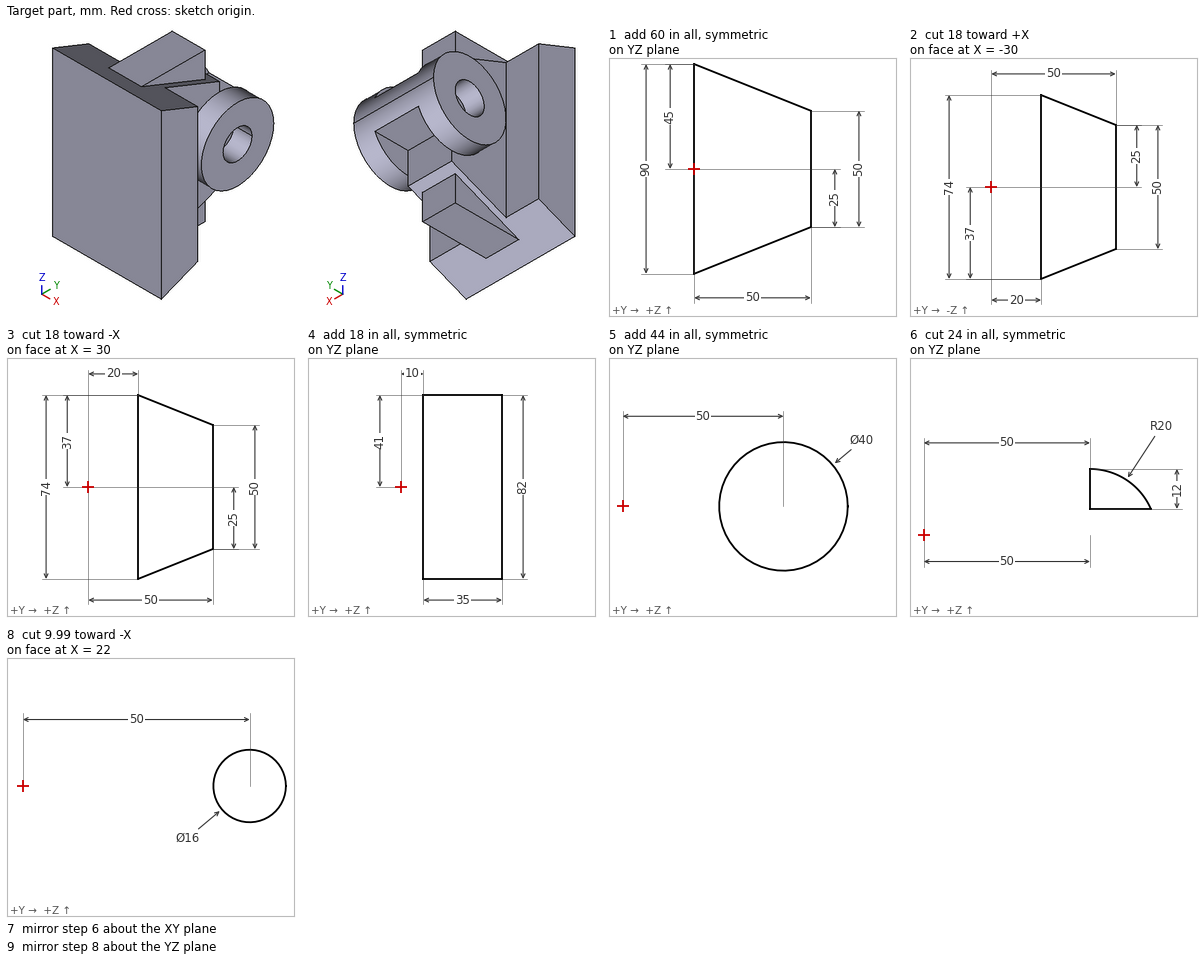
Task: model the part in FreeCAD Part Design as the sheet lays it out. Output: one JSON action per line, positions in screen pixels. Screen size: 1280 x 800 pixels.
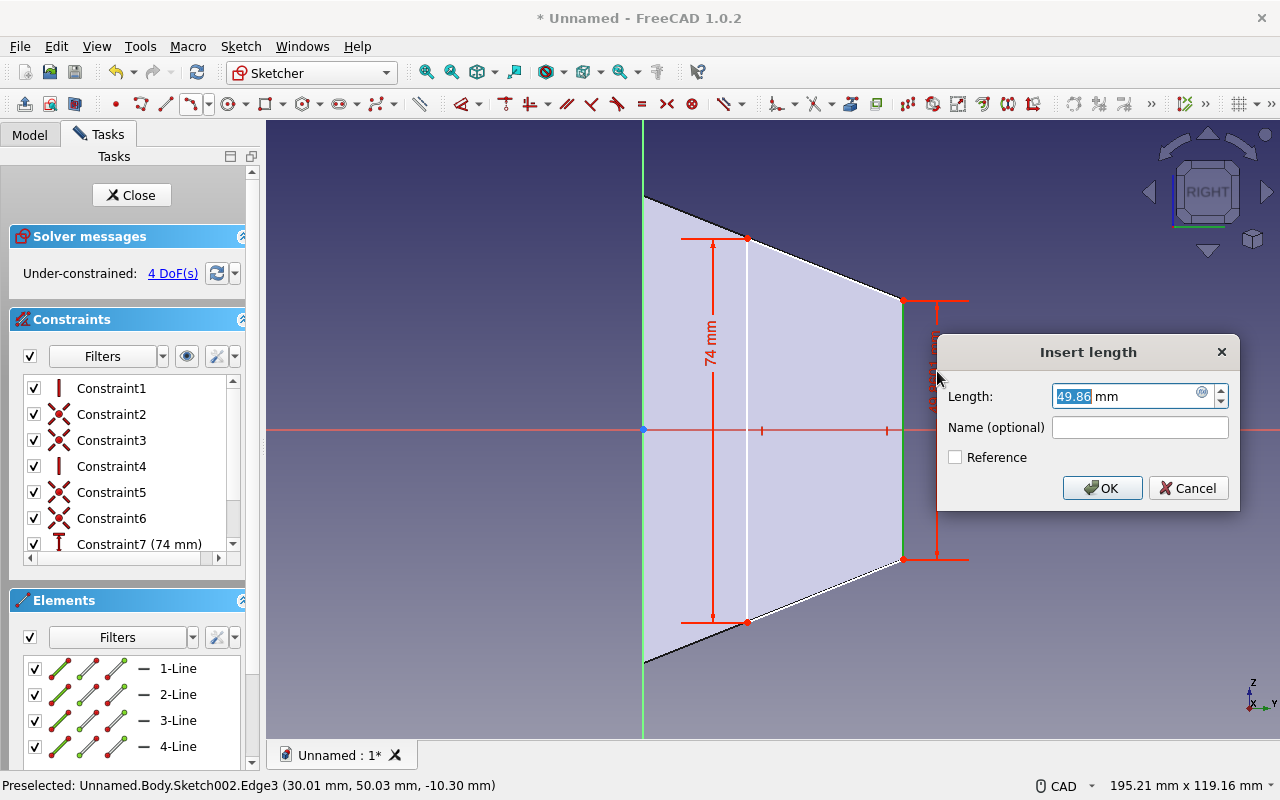
{"action": "type", "text": "50"}
{"action": "key", "text": "Return"}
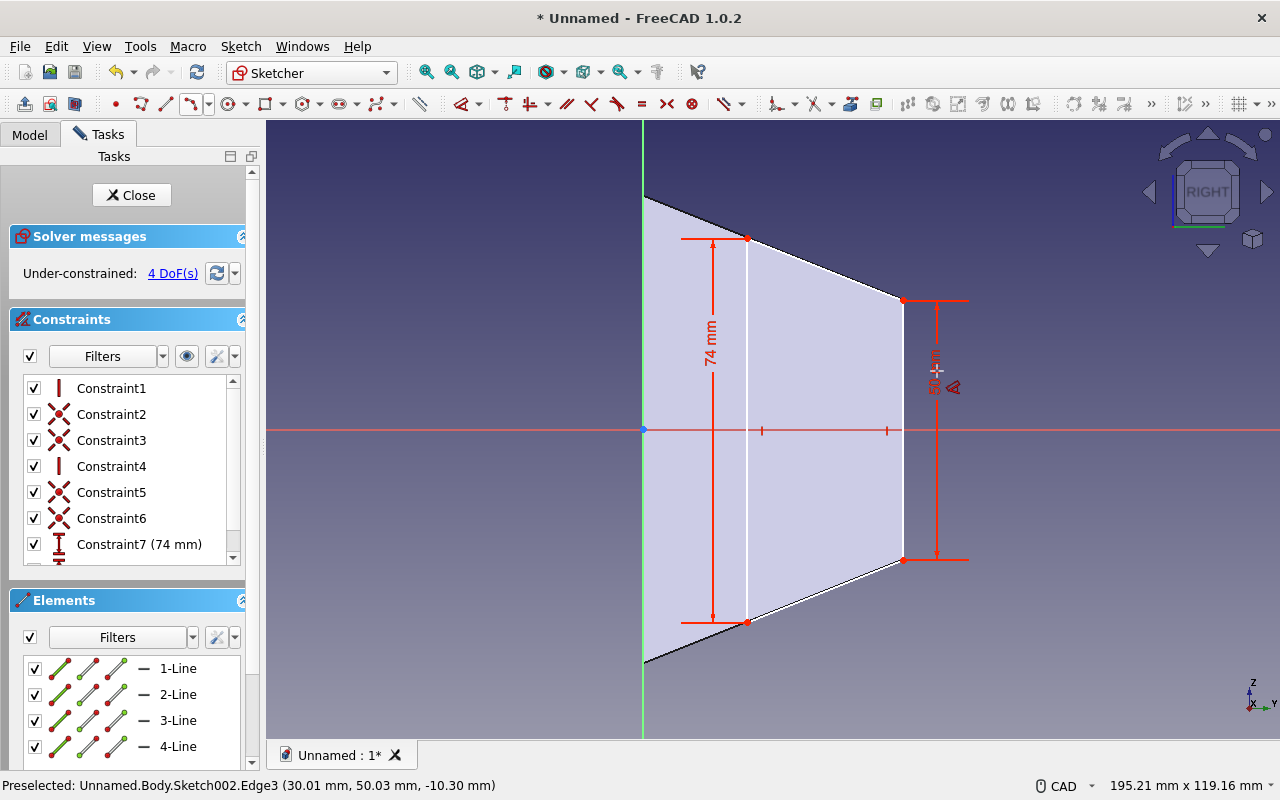
{"action": "left_click", "coordinate": [747, 239]}
{"action": "left_click", "coordinate": [695, 205]}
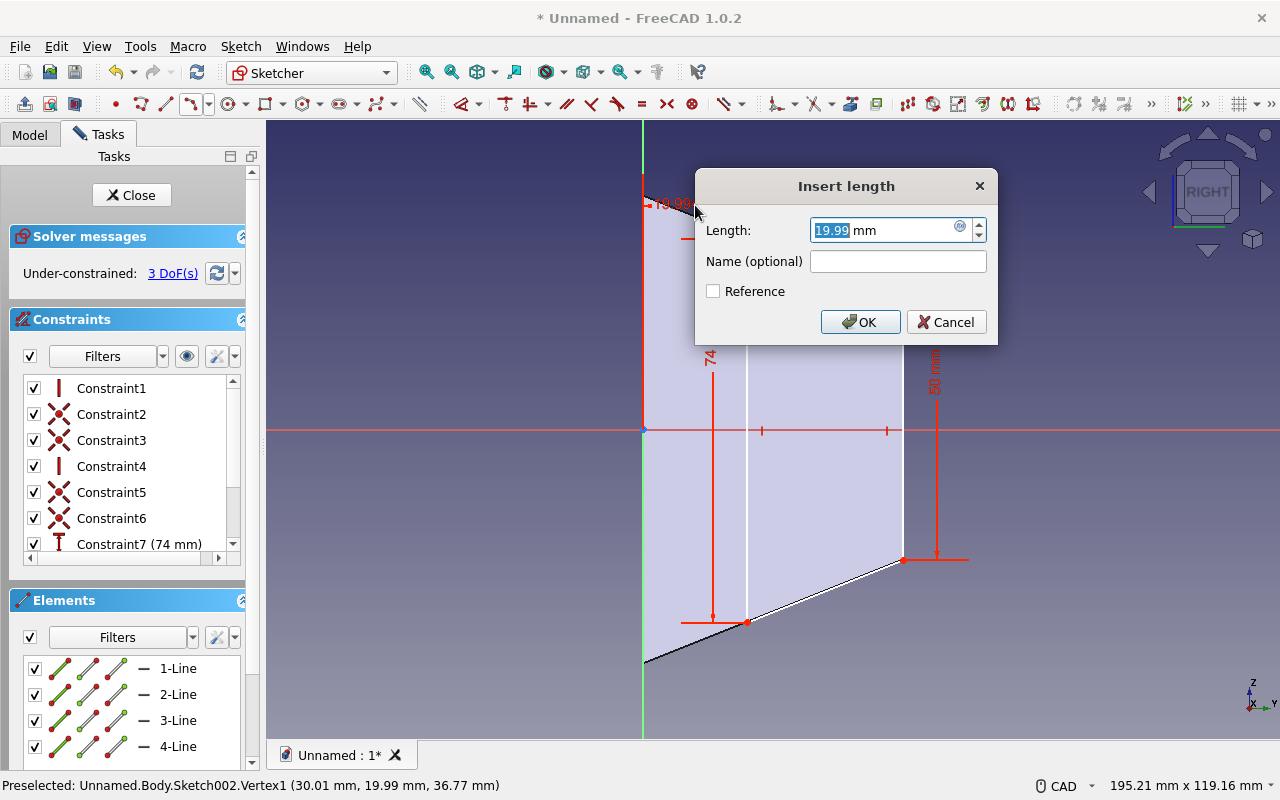
{"action": "type", "text": "20"}
{"action": "key", "text": "Return"}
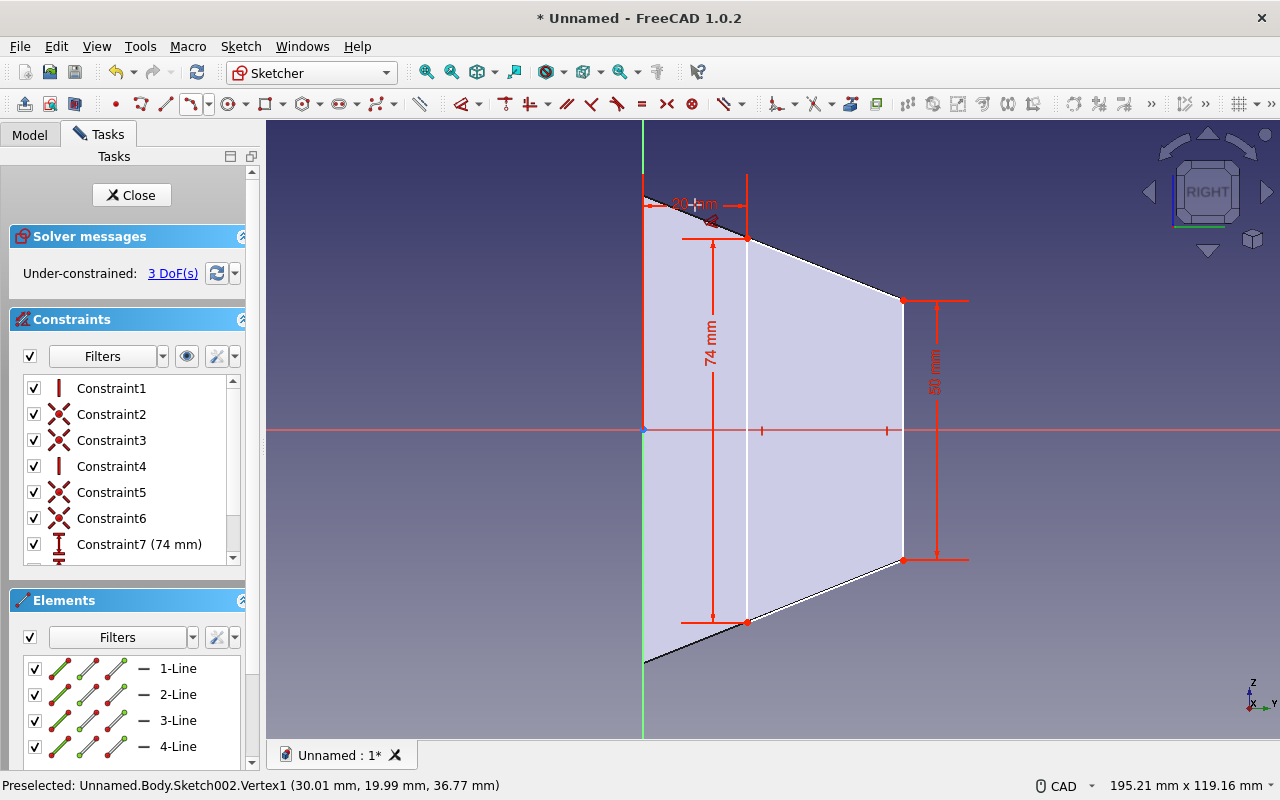
{"action": "left_click", "coordinate": [747, 239]}
{"action": "left_click", "coordinate": [609, 334]}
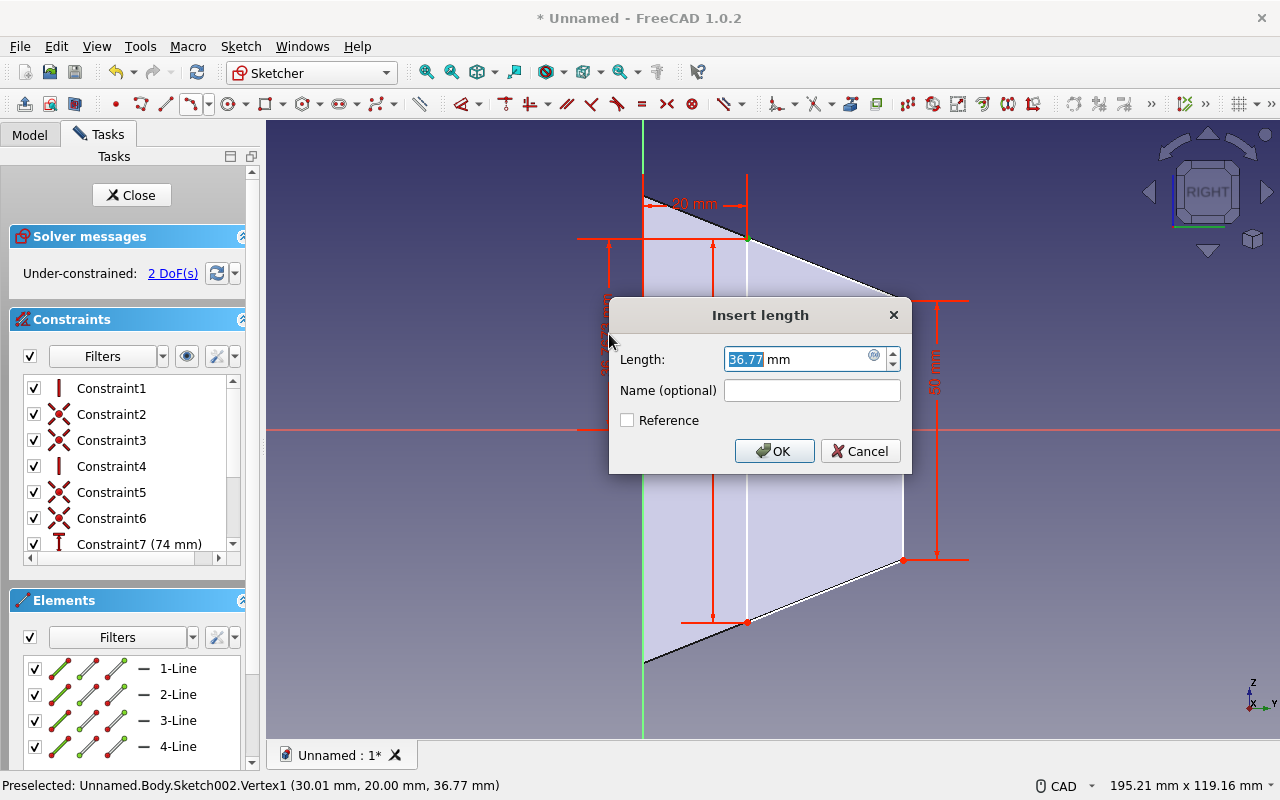
{"action": "type", "text": "37"}
{"action": "key", "text": "Return"}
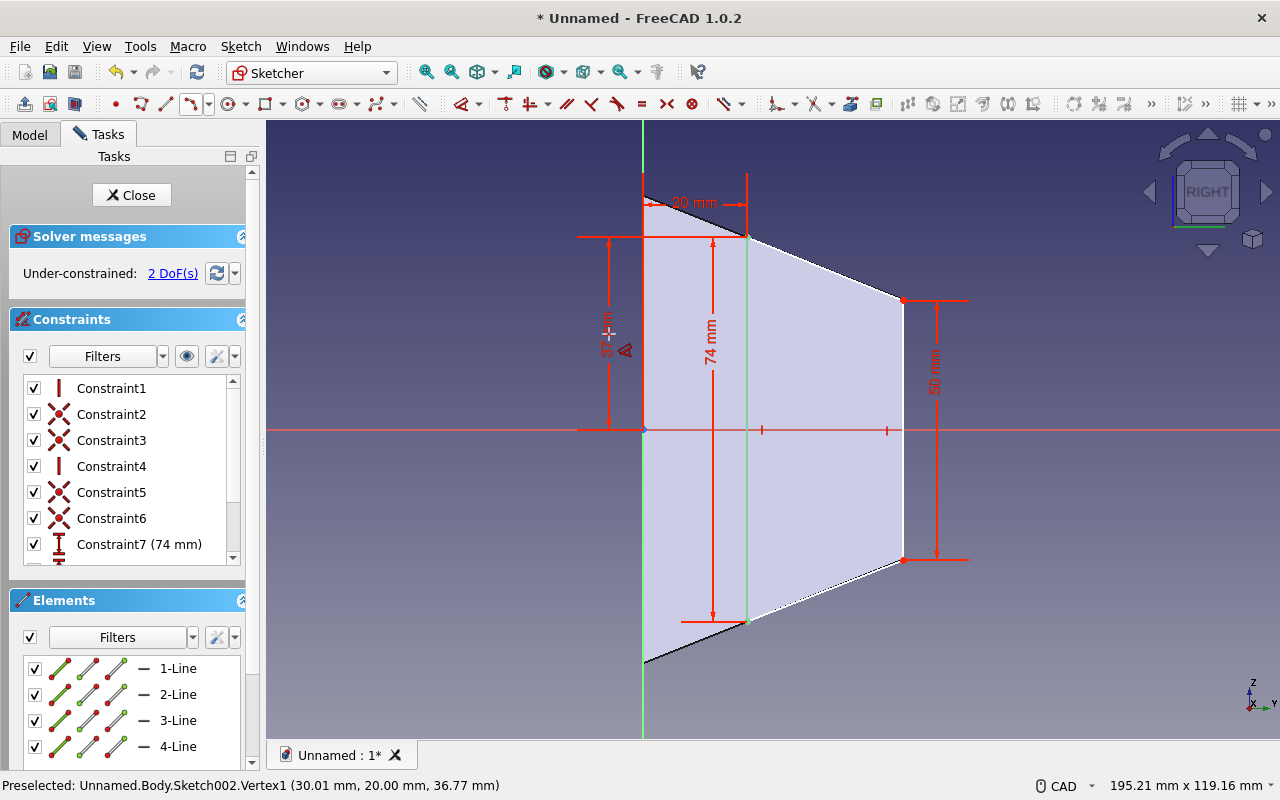
{"action": "left_click", "coordinate": [903, 560]}
{"action": "left_click", "coordinate": [773, 594]}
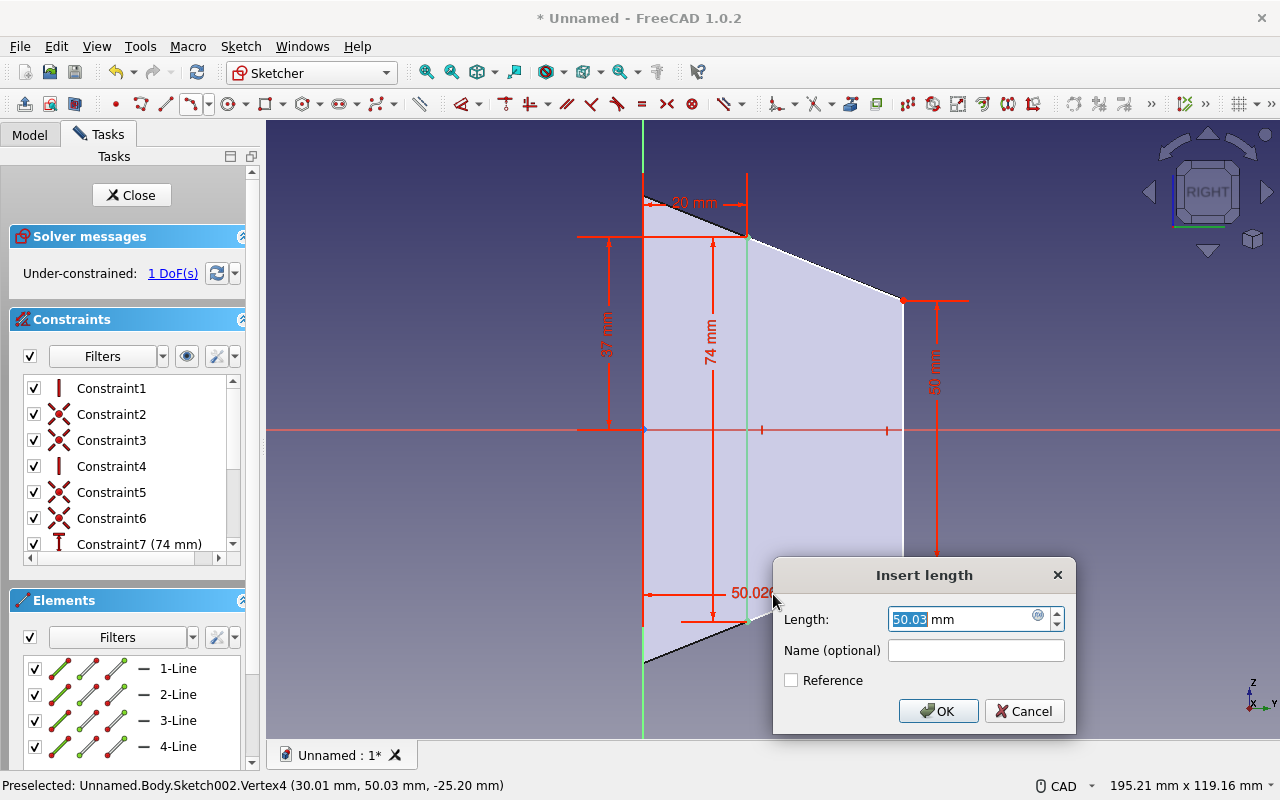
{"action": "type", "text": "50"}
{"action": "key", "text": "Return"}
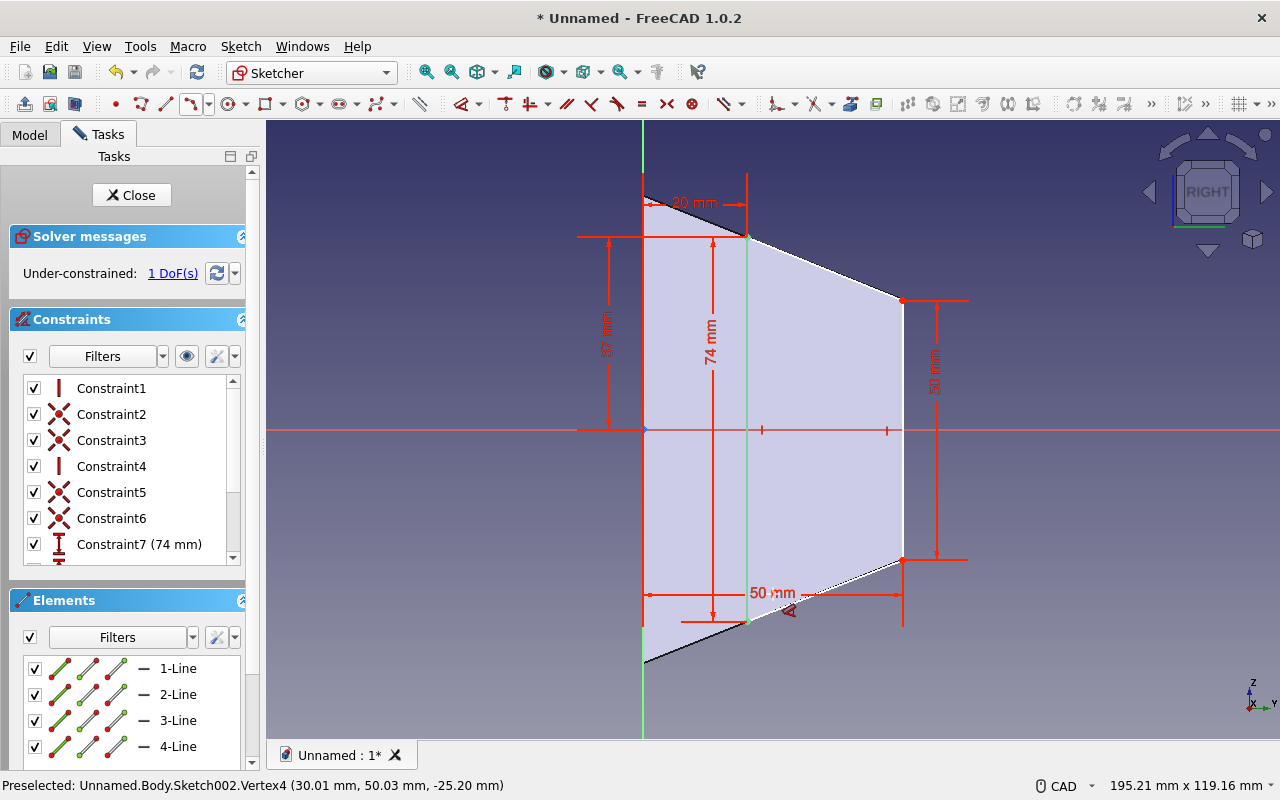
{"action": "left_click", "coordinate": [903, 560]}
{"action": "left_click", "coordinate": [937, 495]}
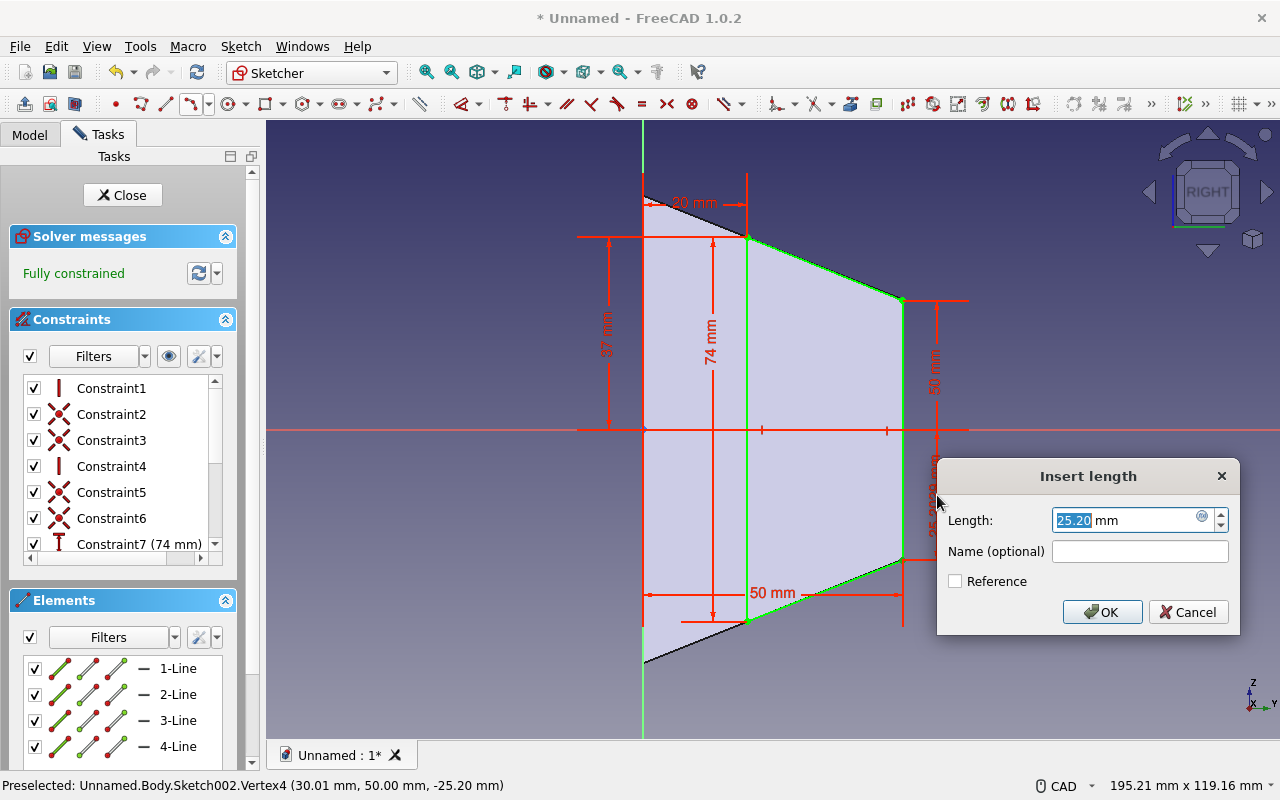
{"action": "type", "text": "25"}
{"action": "key", "text": "Return"}
{"action": "key", "text": "Escape"}